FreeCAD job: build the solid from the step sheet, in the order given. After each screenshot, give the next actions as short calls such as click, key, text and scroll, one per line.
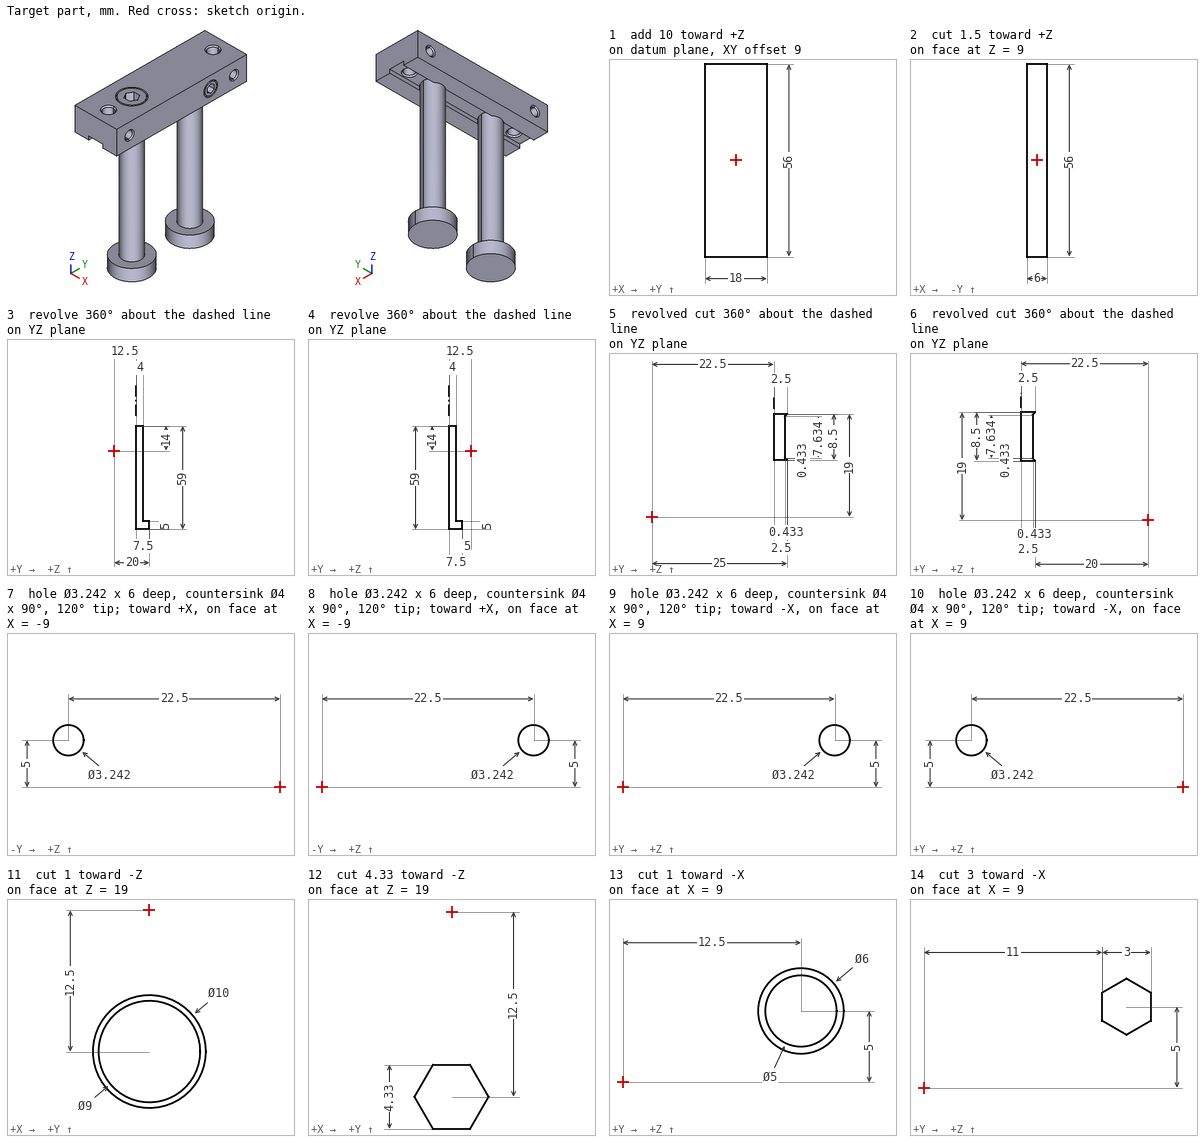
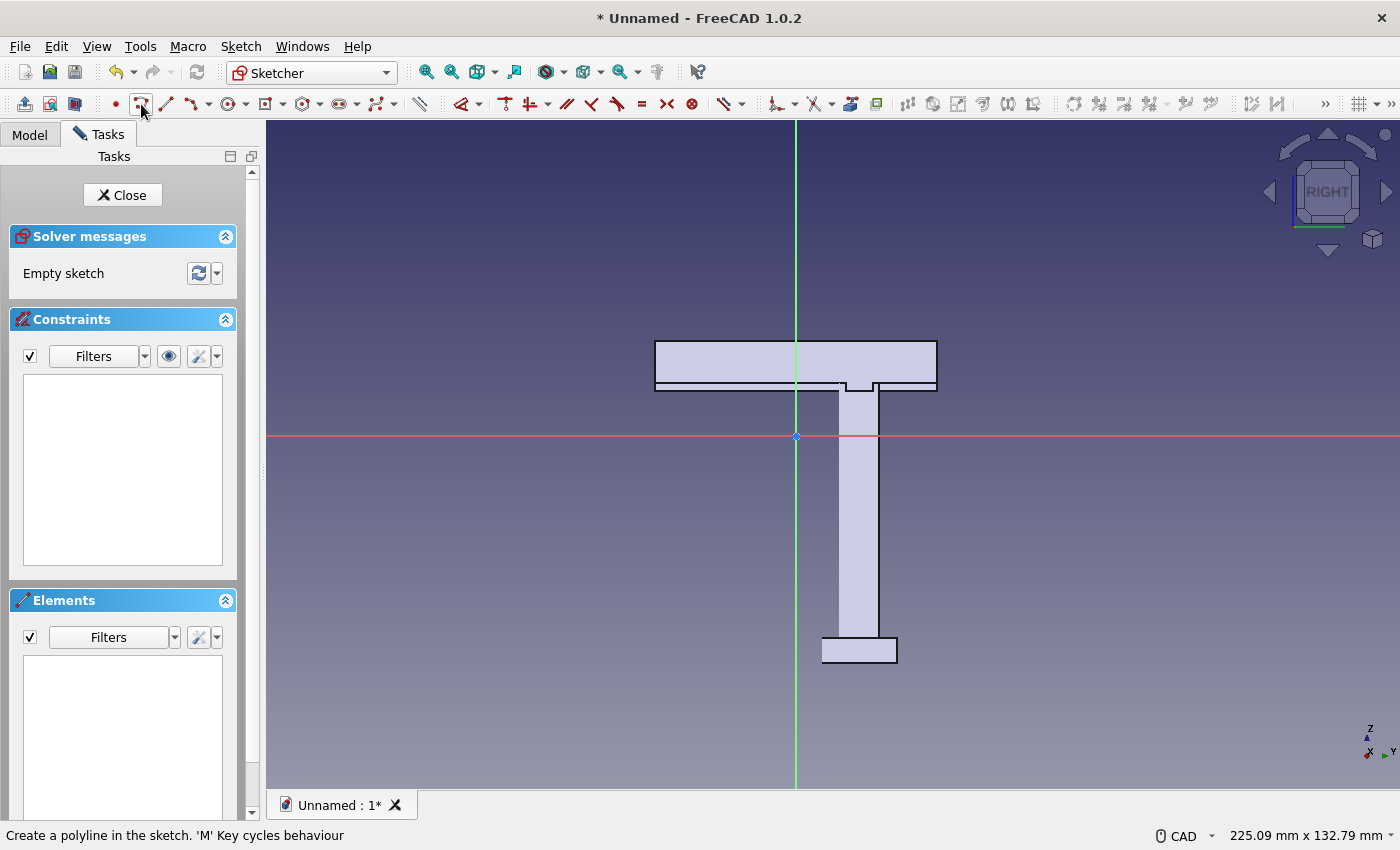
click(754, 366)
click(733, 366)
click(733, 663)
click(771, 663)
click(771, 638)
click(754, 638)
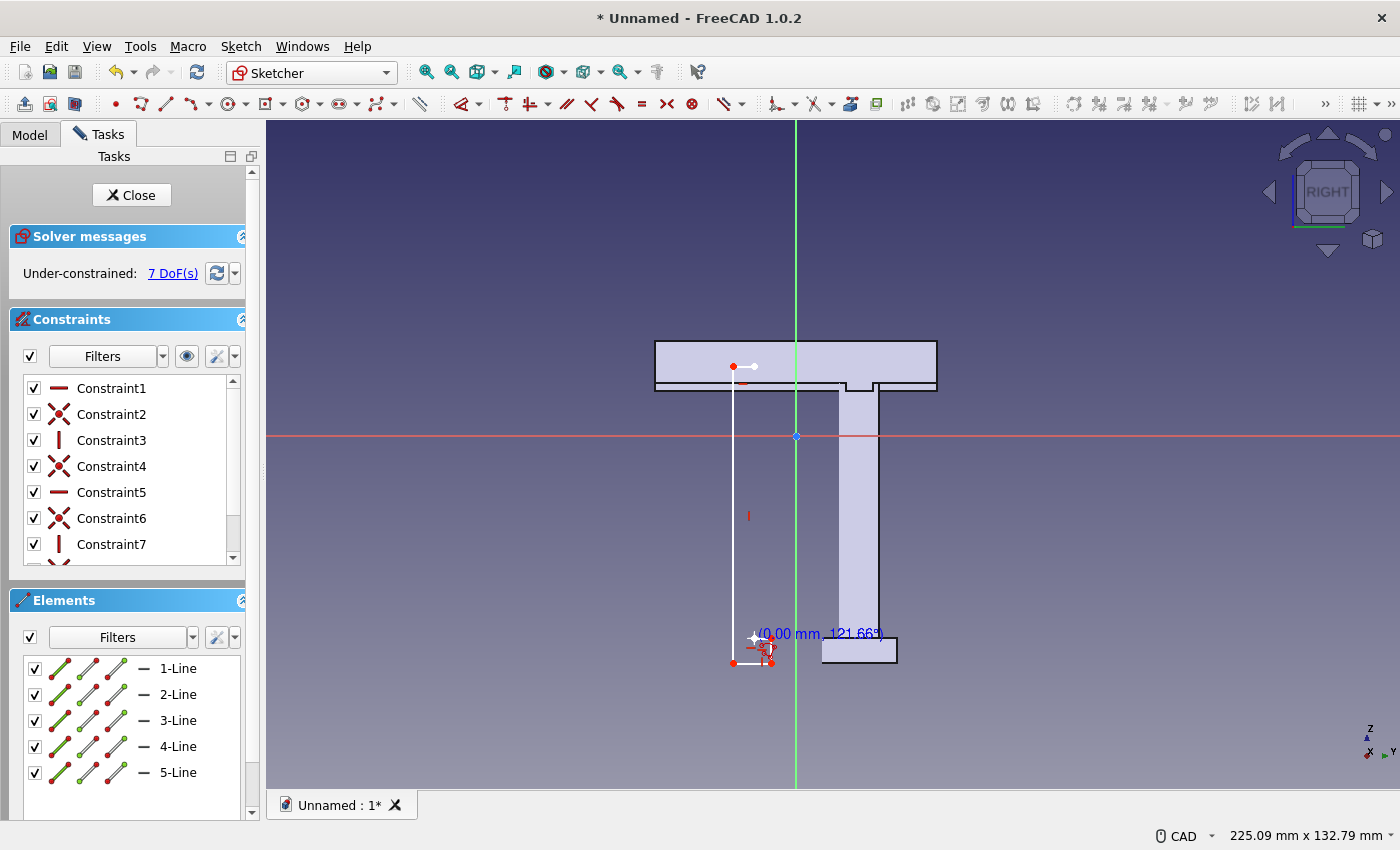
scroll(754, 366, up, 3)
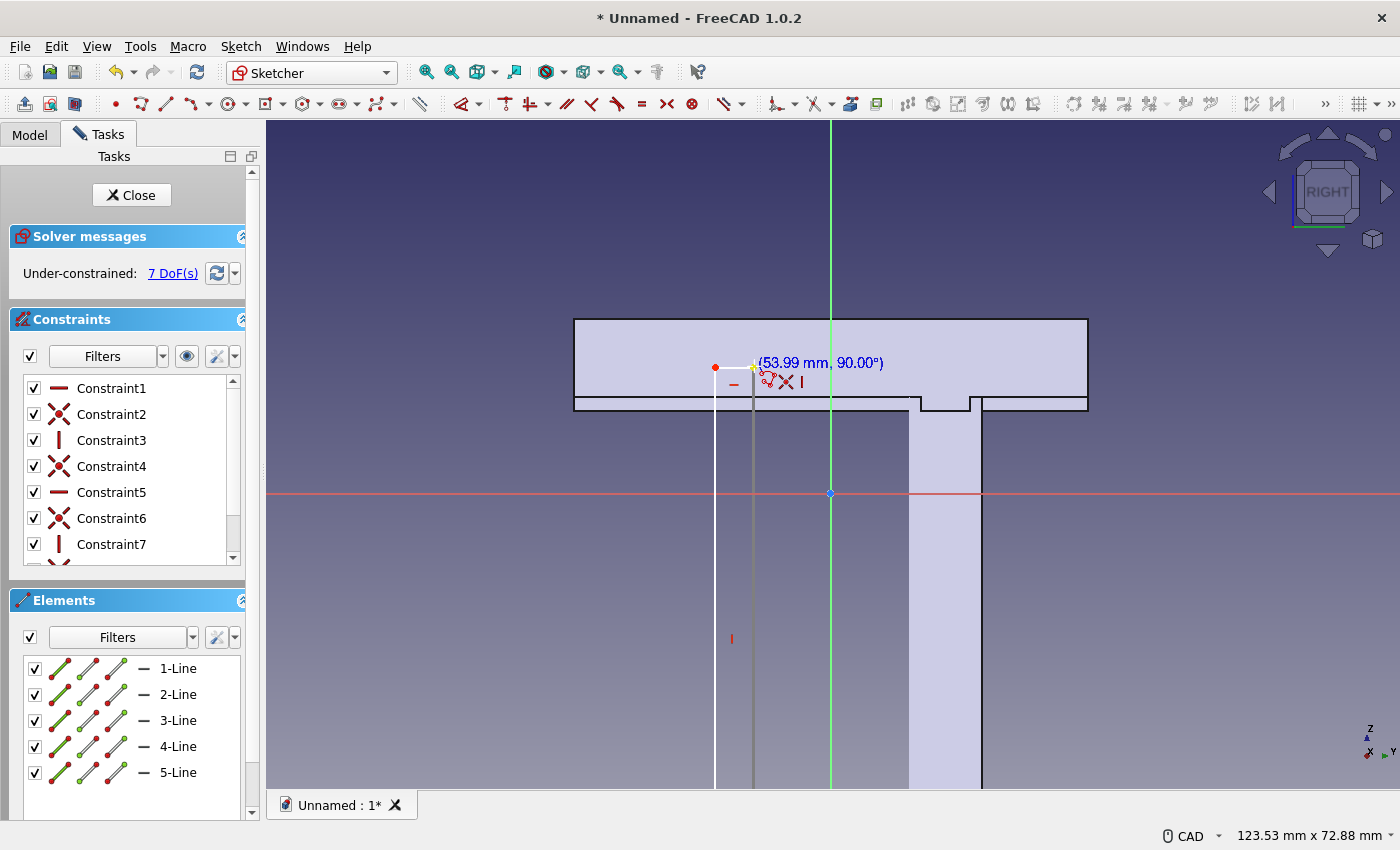
click(754, 368)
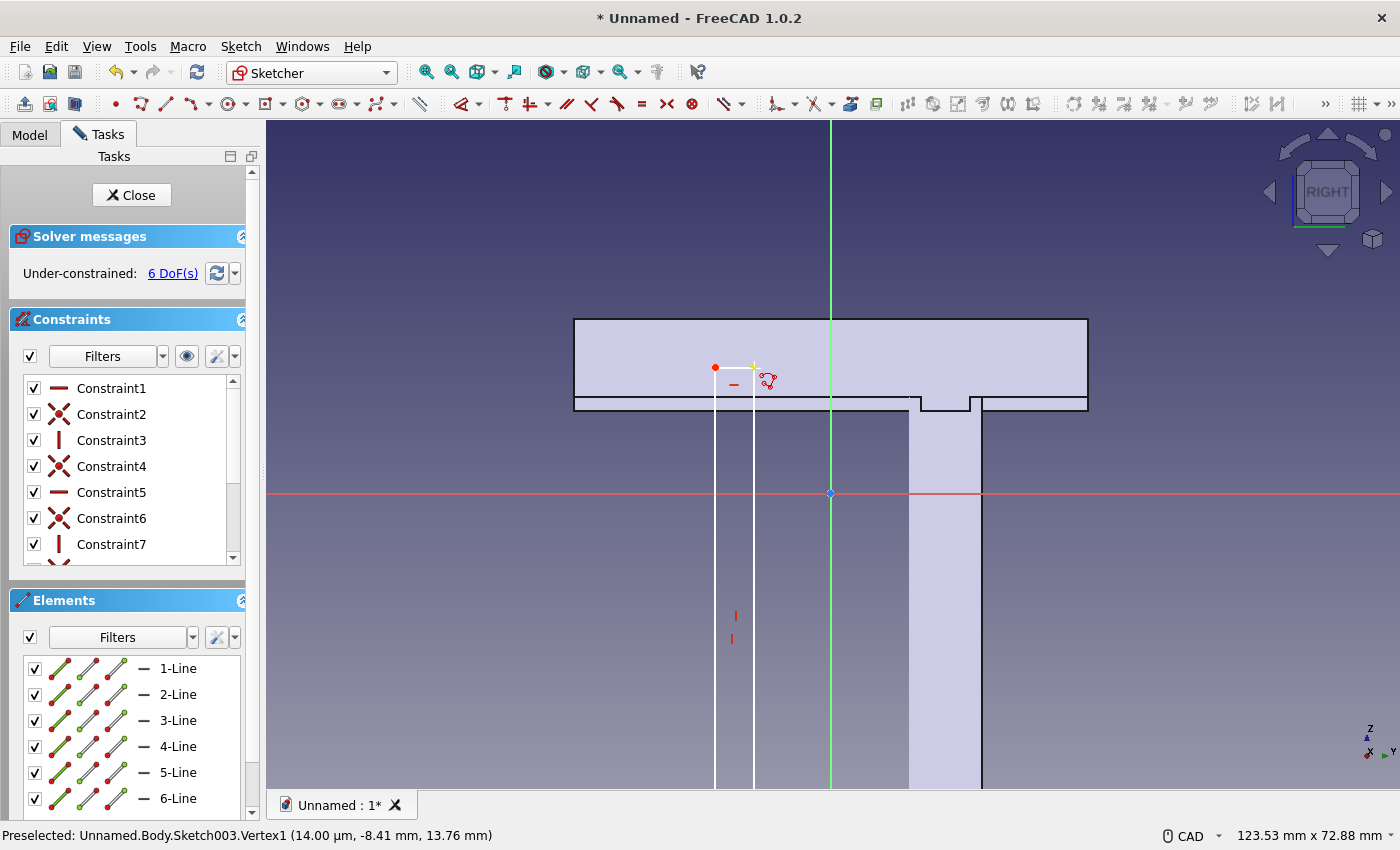
click(166, 104)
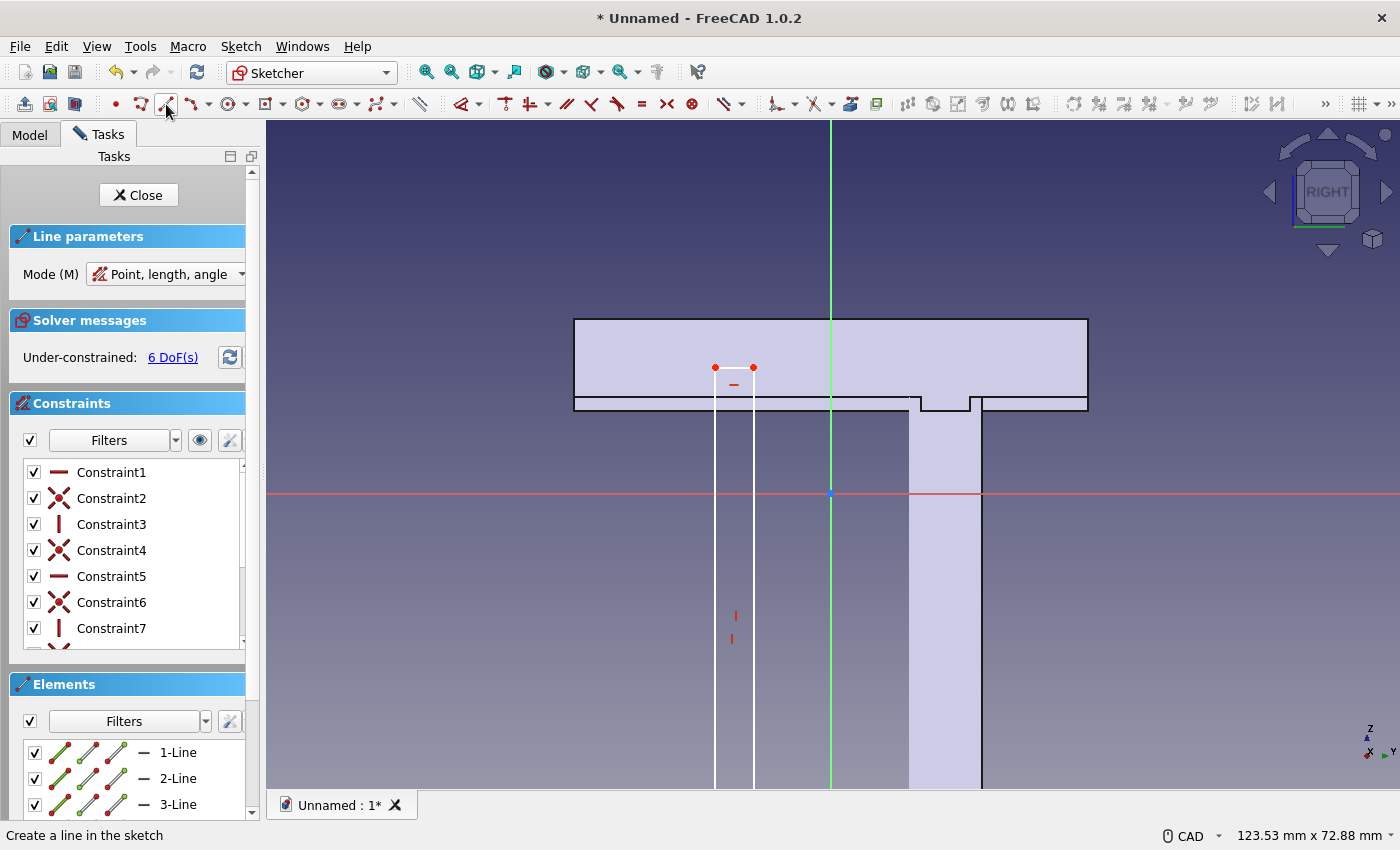
click(716, 311)
click(716, 149)
key(Escape)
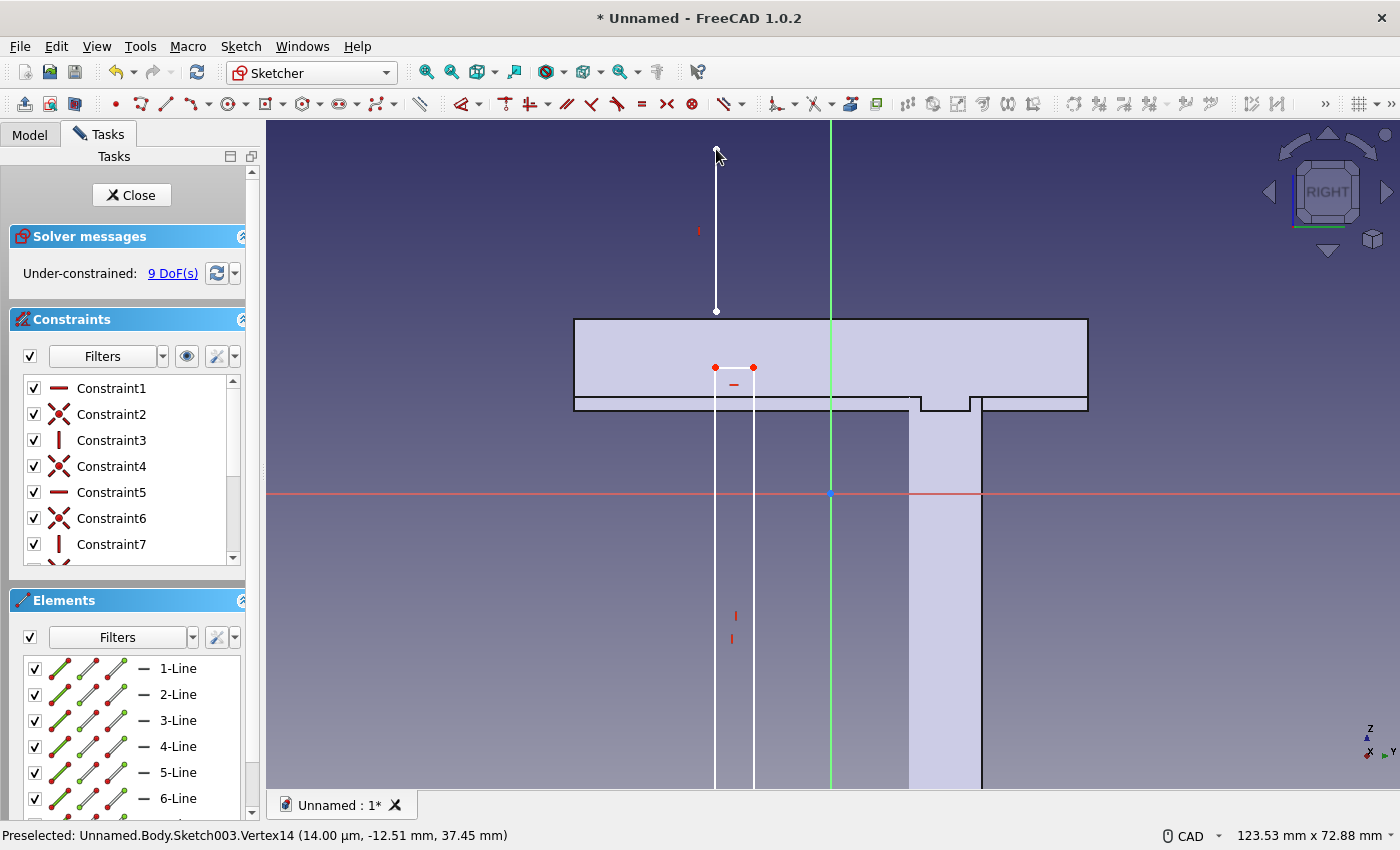
click(716, 263)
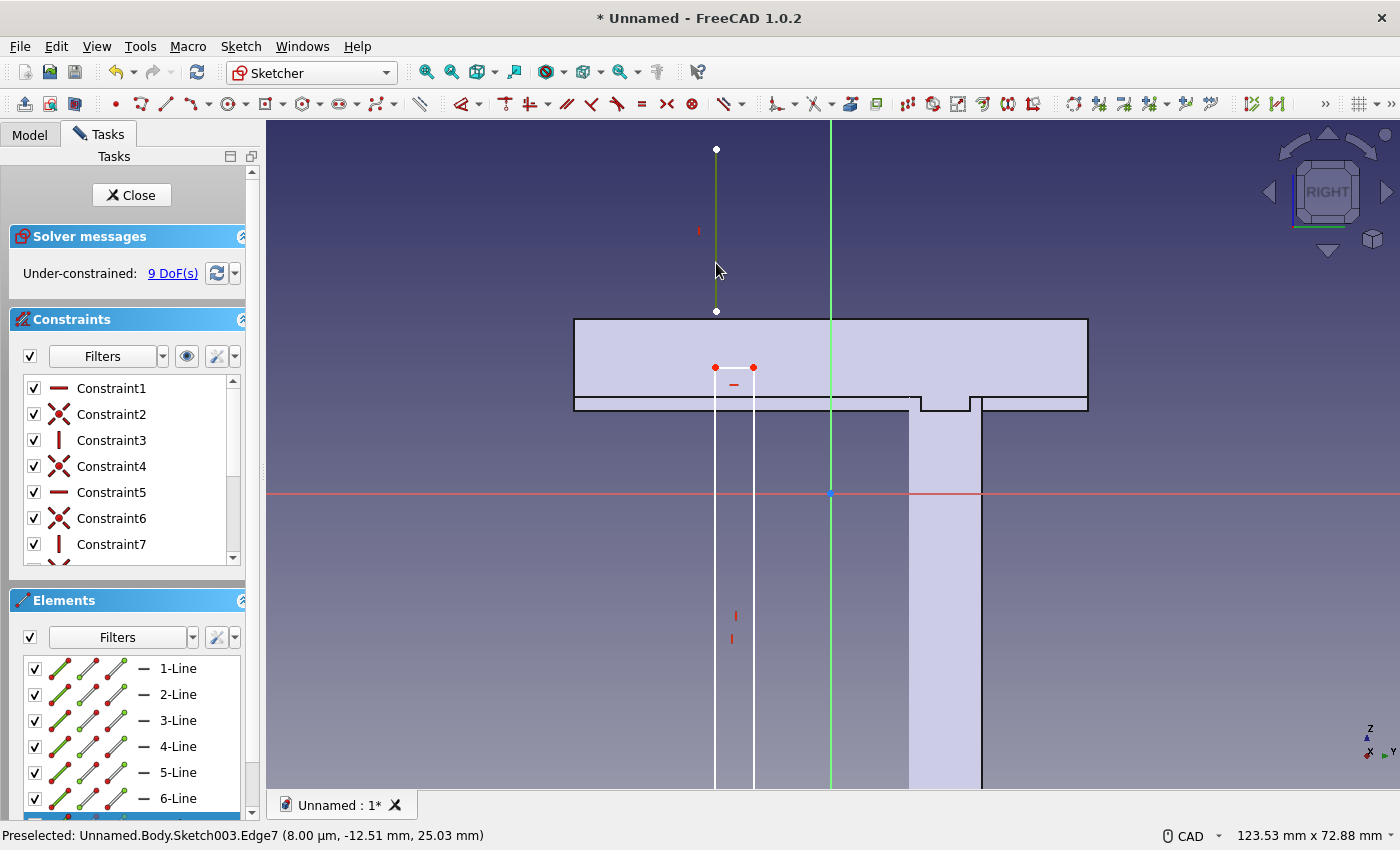
click(420, 104)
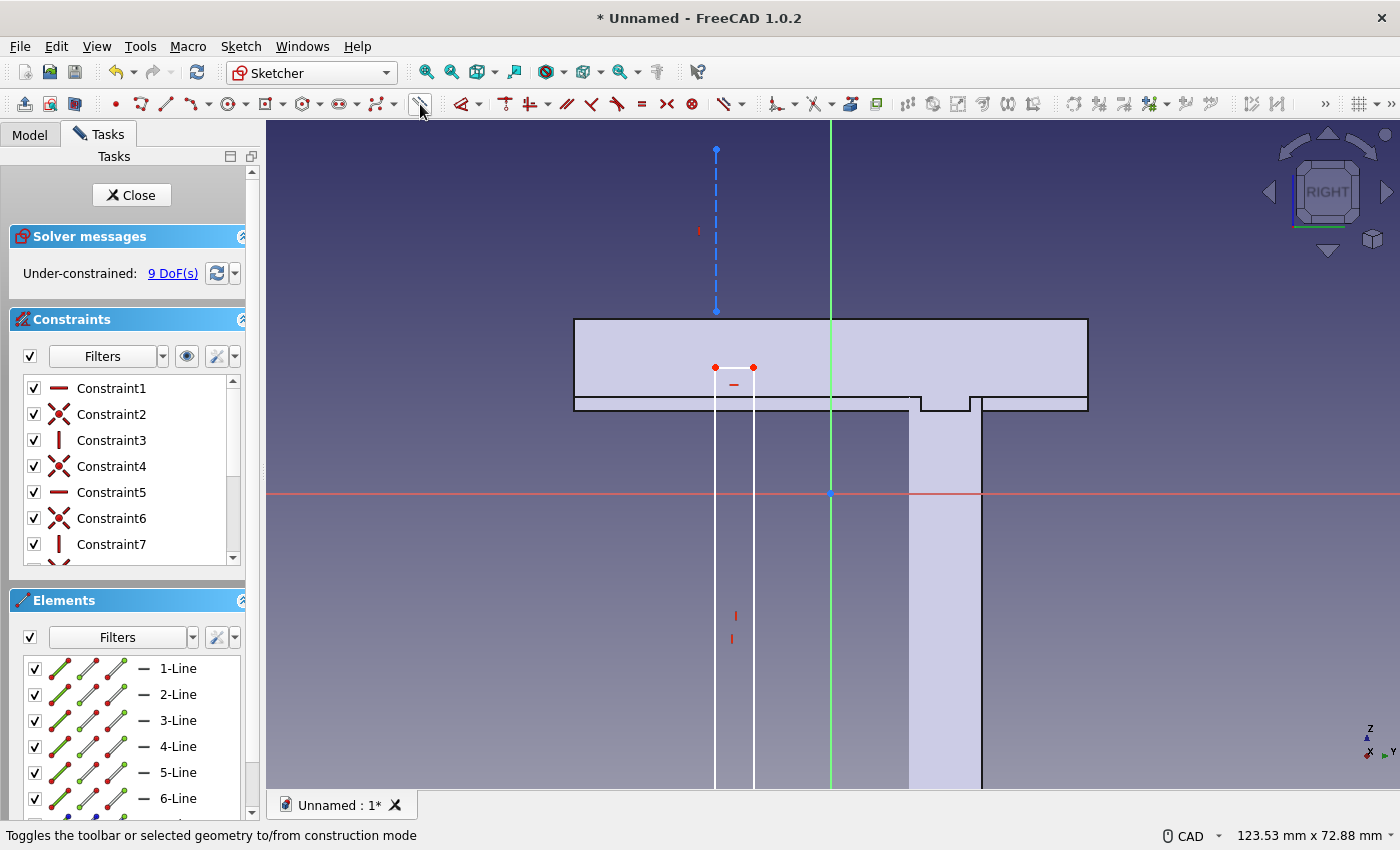
click(460, 104)